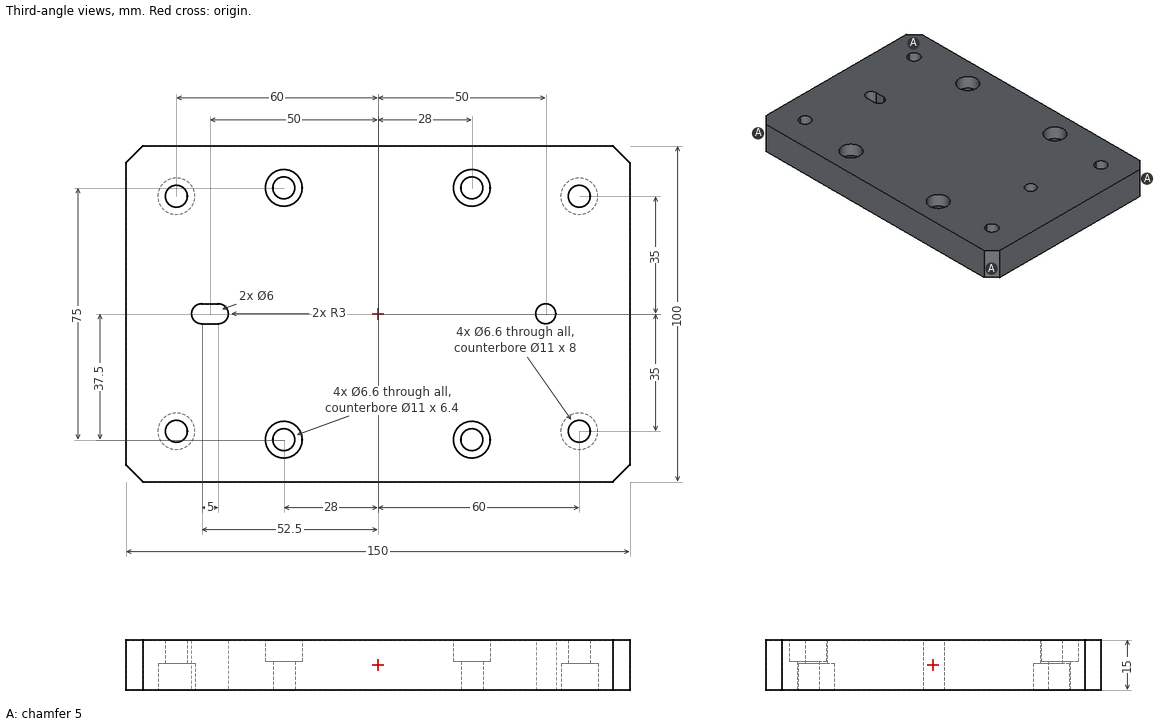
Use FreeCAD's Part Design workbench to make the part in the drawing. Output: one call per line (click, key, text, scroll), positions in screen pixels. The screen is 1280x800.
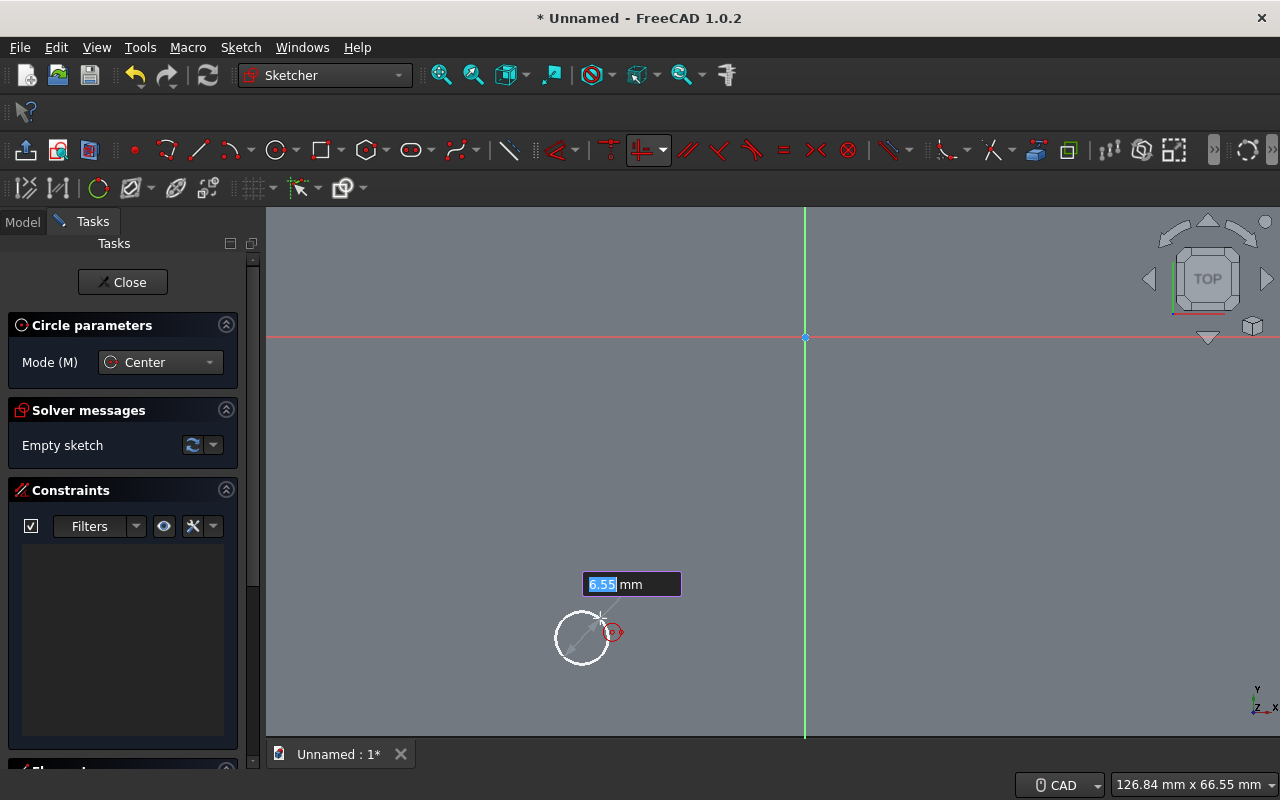
text(6.6)
key(Return)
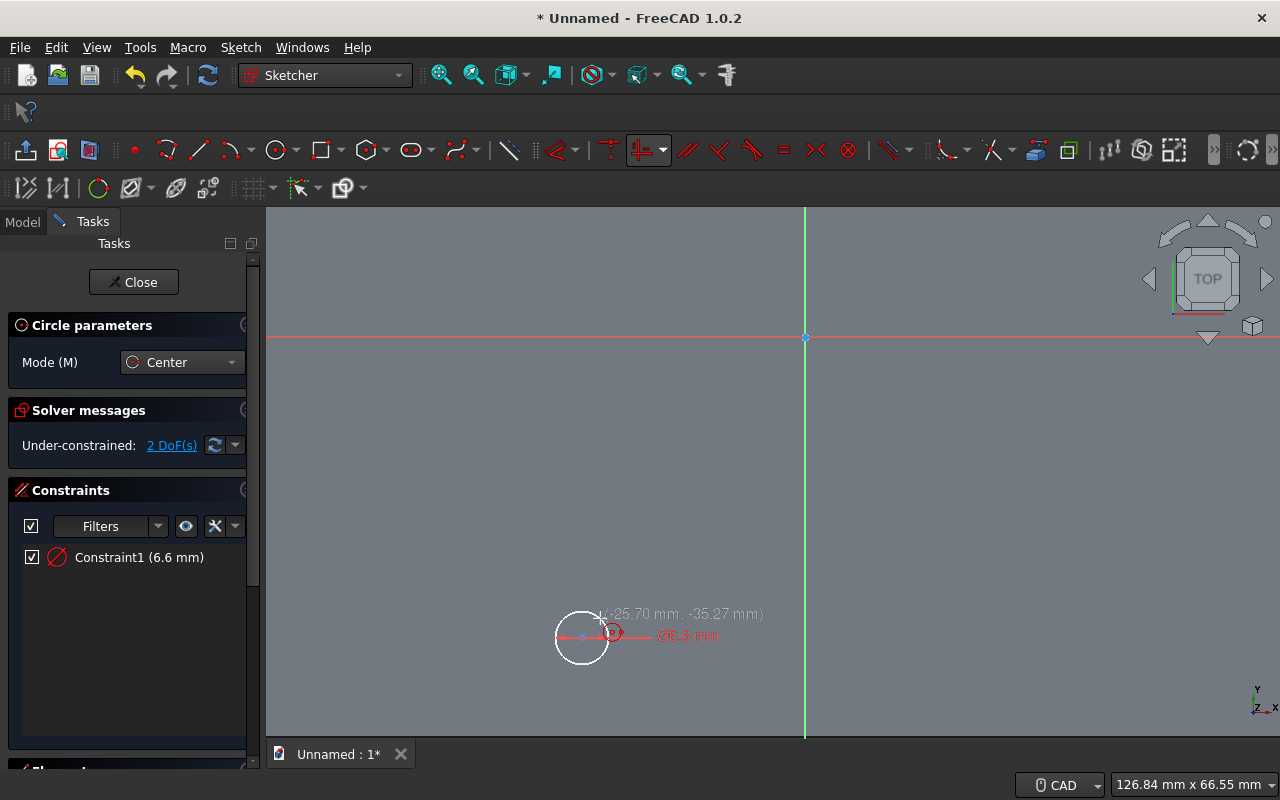
scroll(582, 638, down, 3)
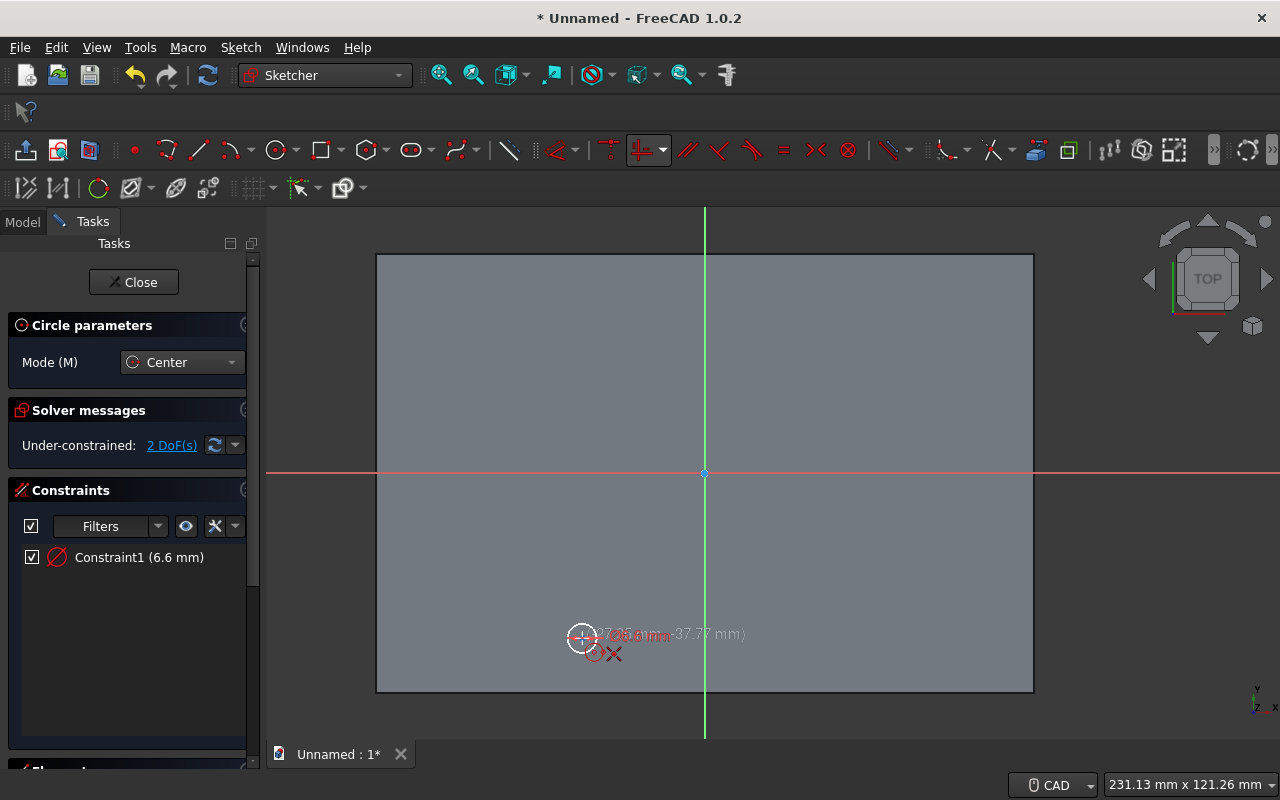
scroll(582, 309, up, 3)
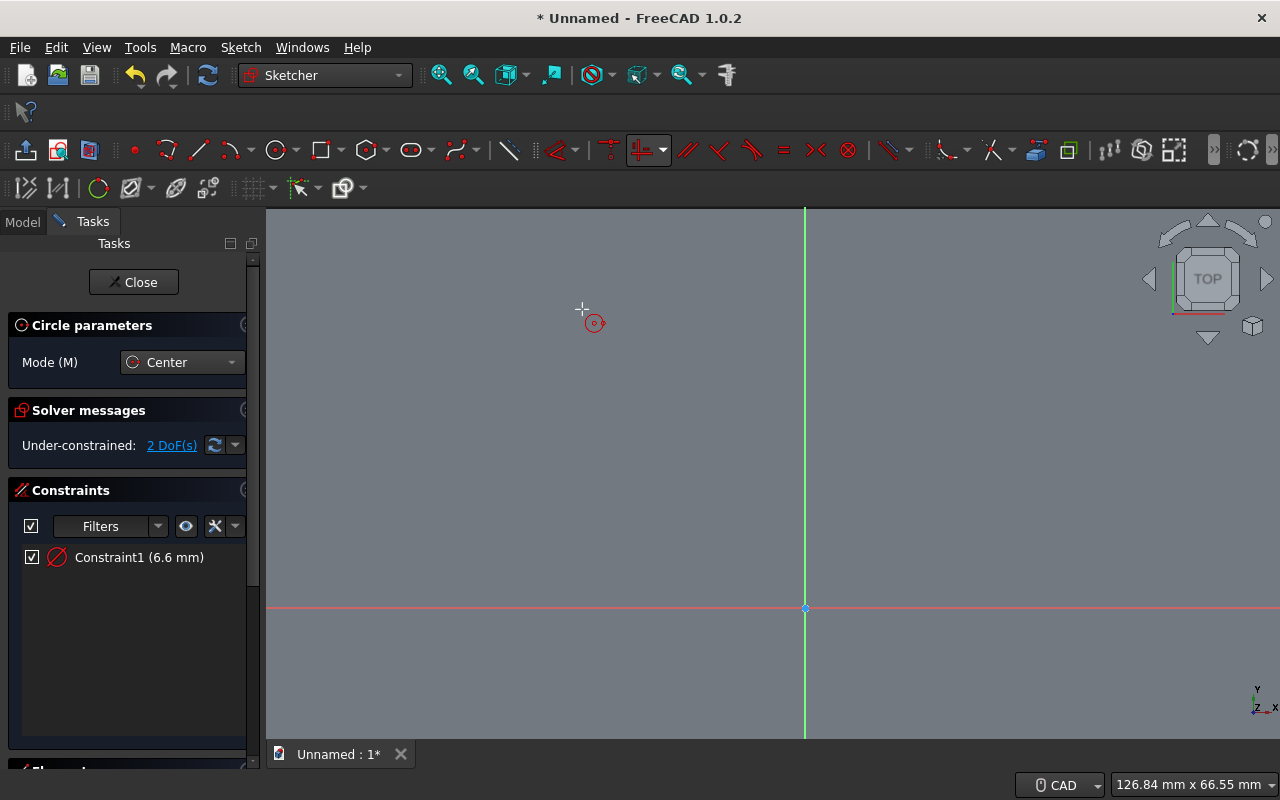
click(582, 308)
move(600, 290)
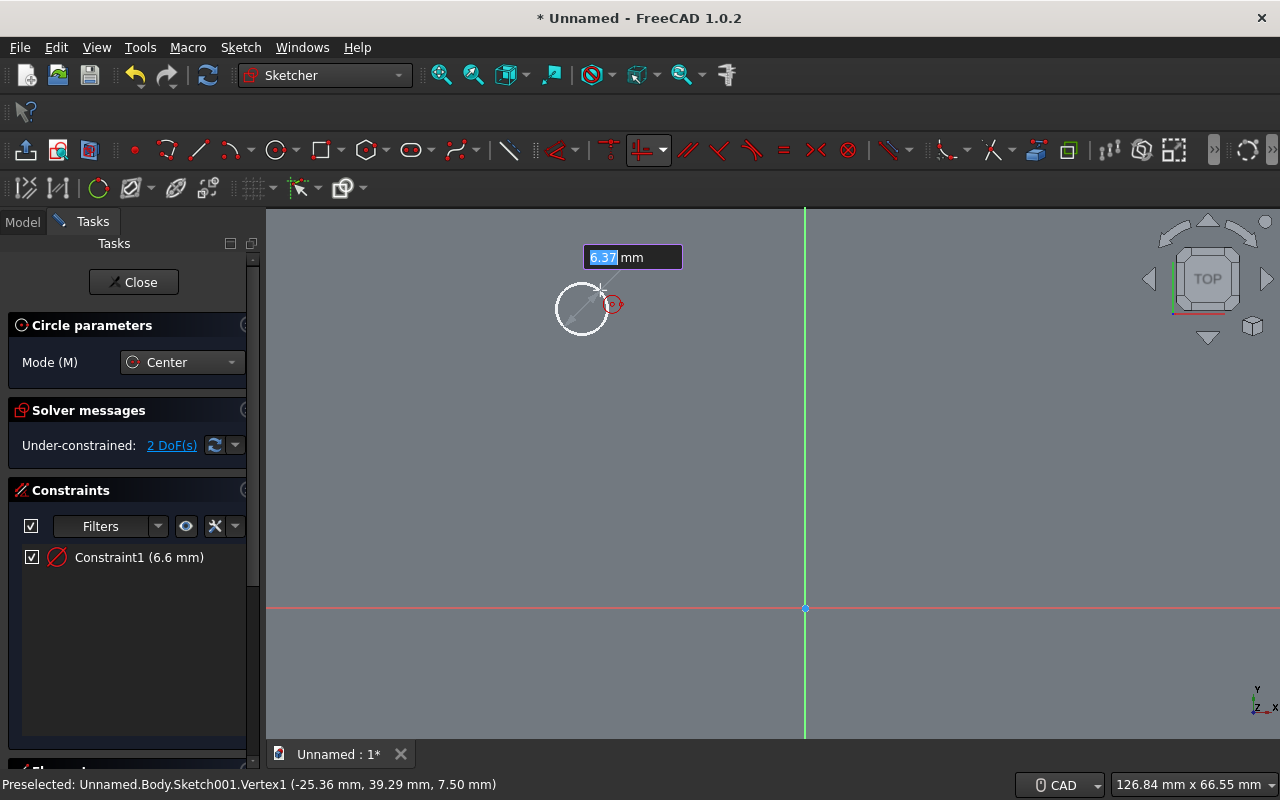
text(6.6)
key(Return)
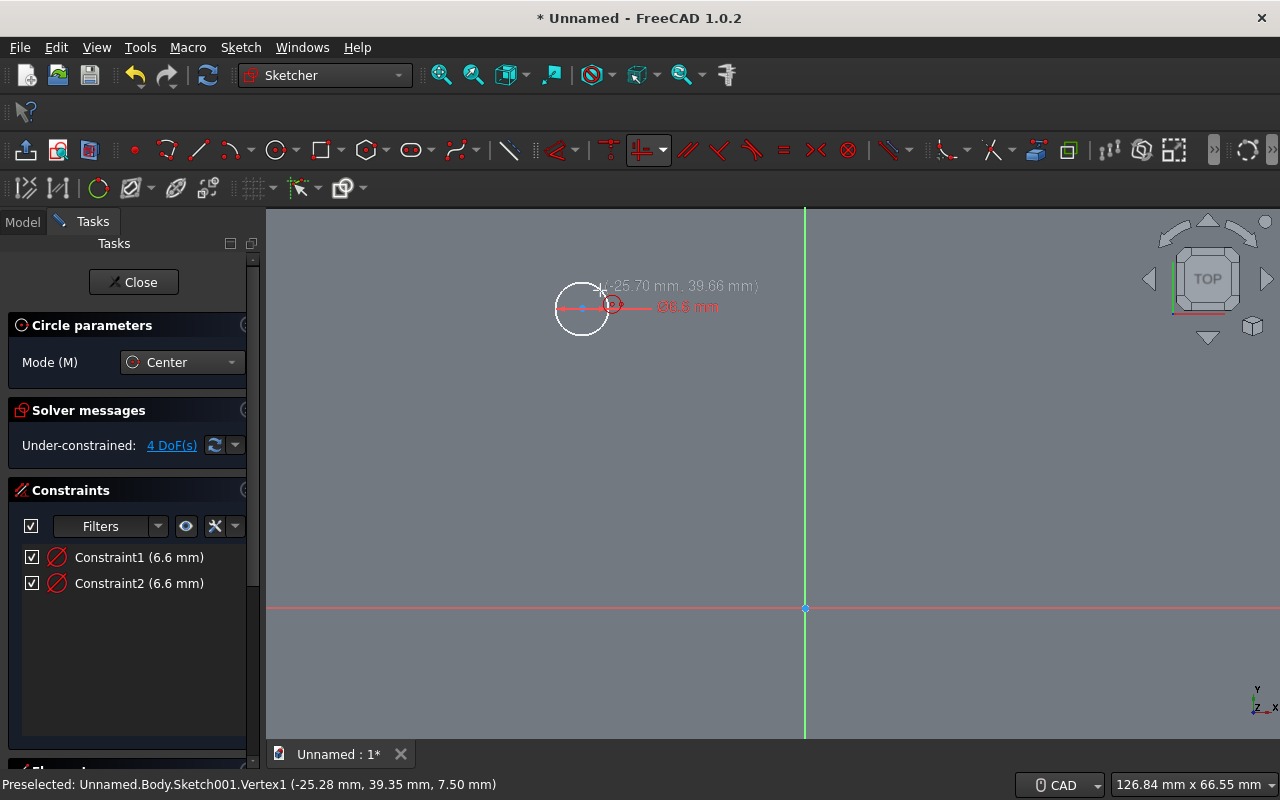
click(1029, 308)
move(1048, 290)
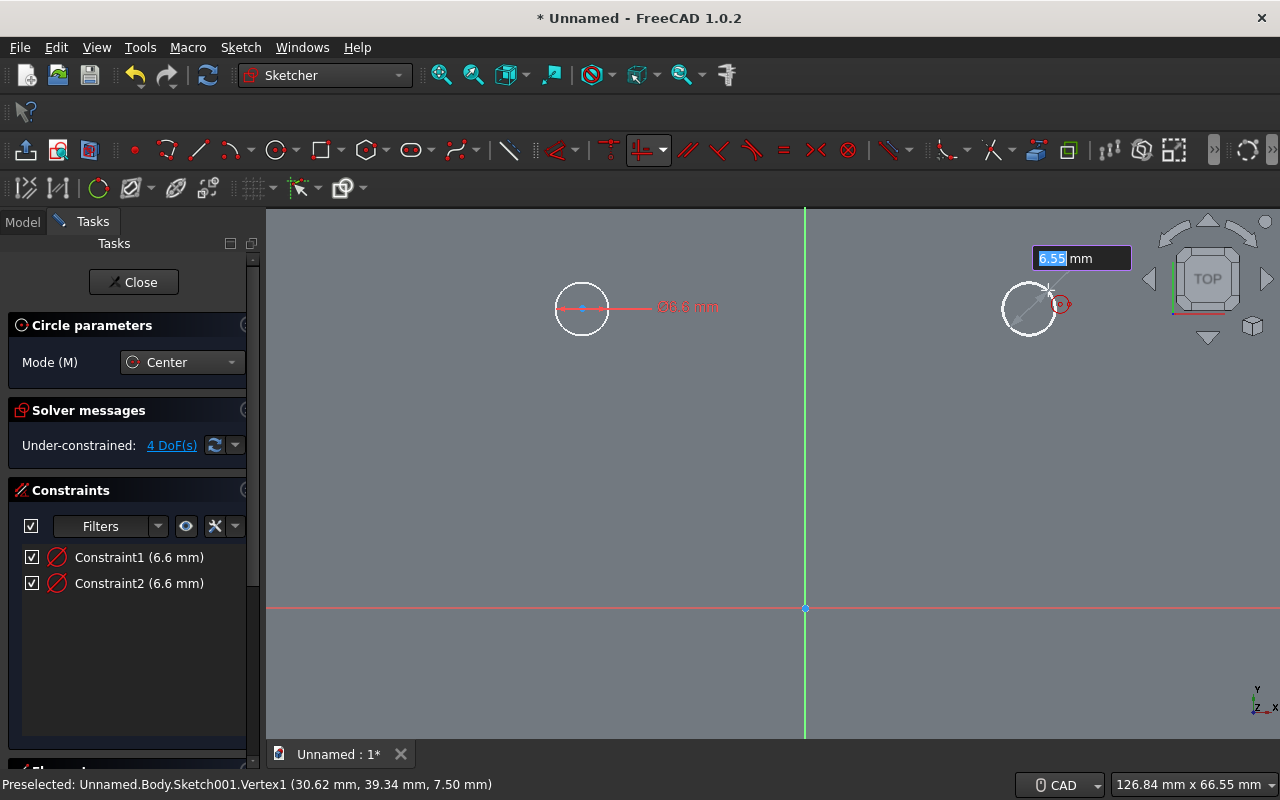
text(6.6)
key(Return)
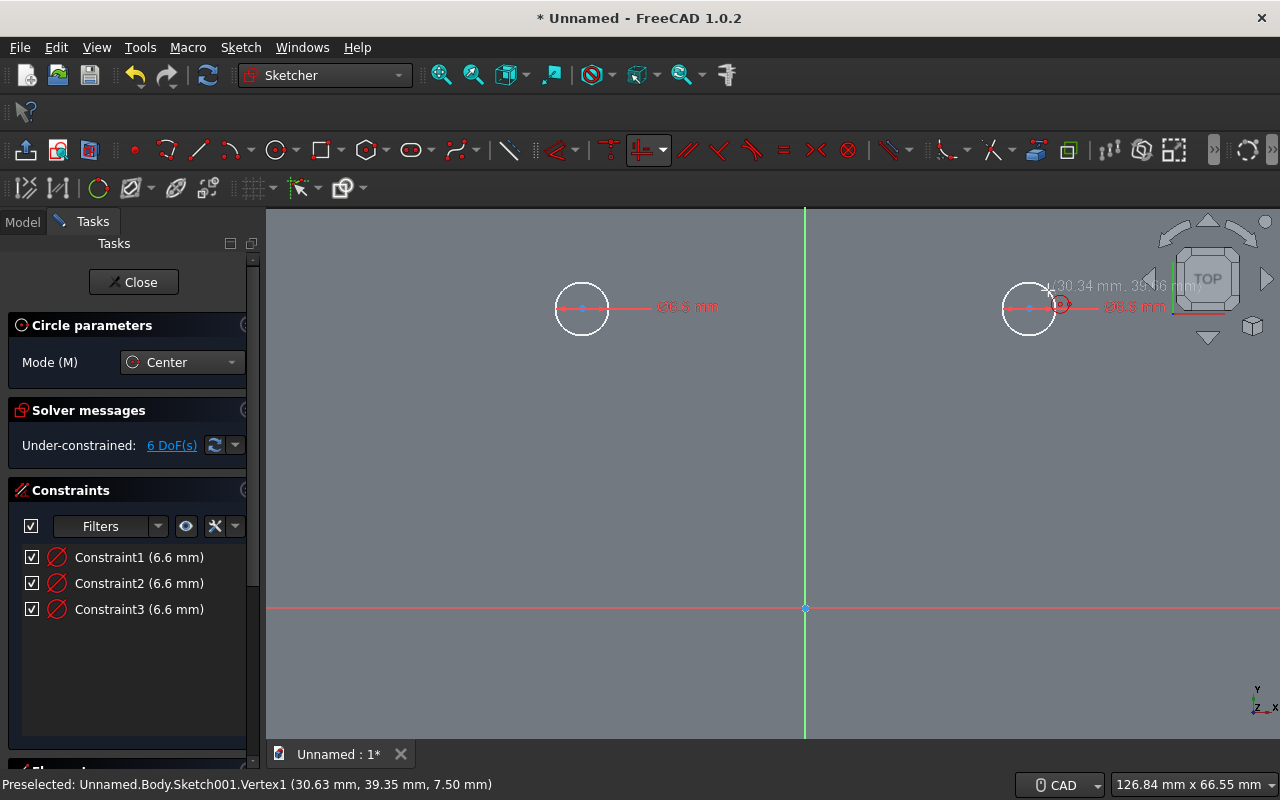
scroll(582, 309, down, 3)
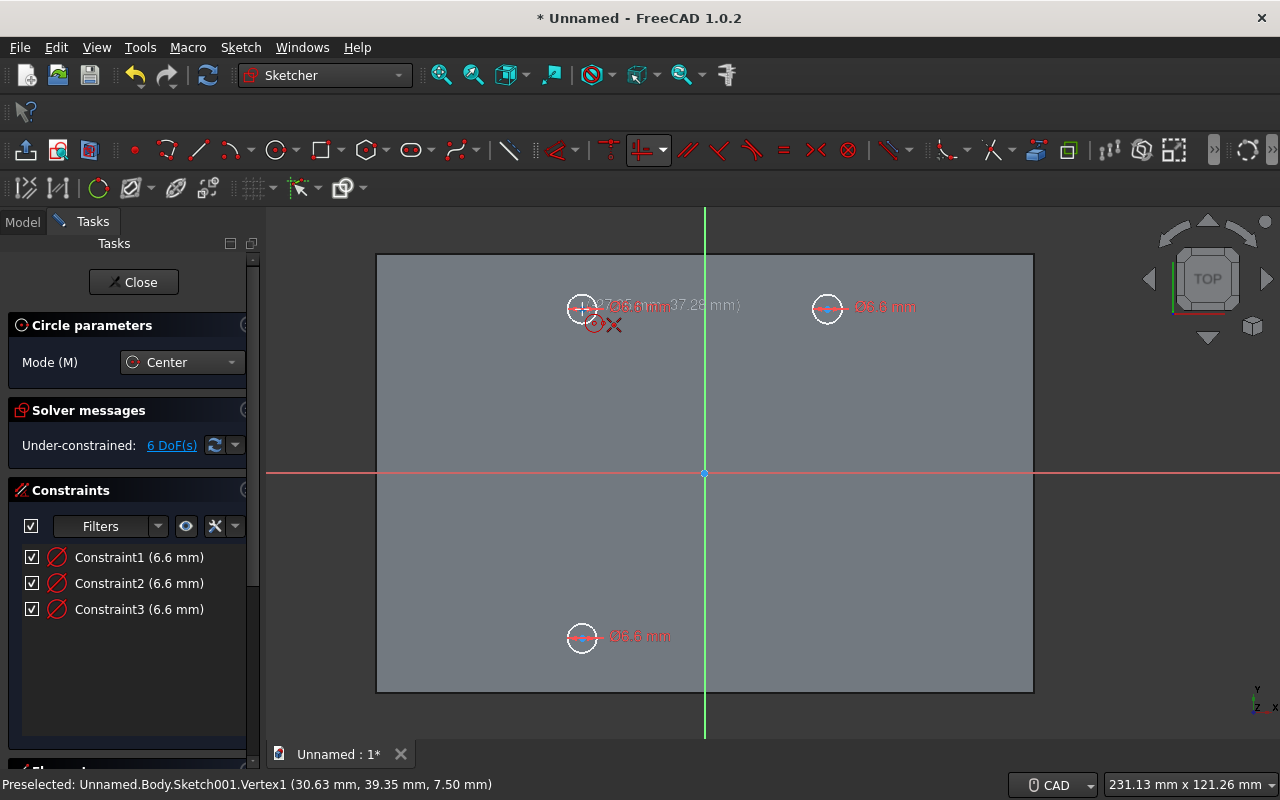
scroll(828, 638, up, 3)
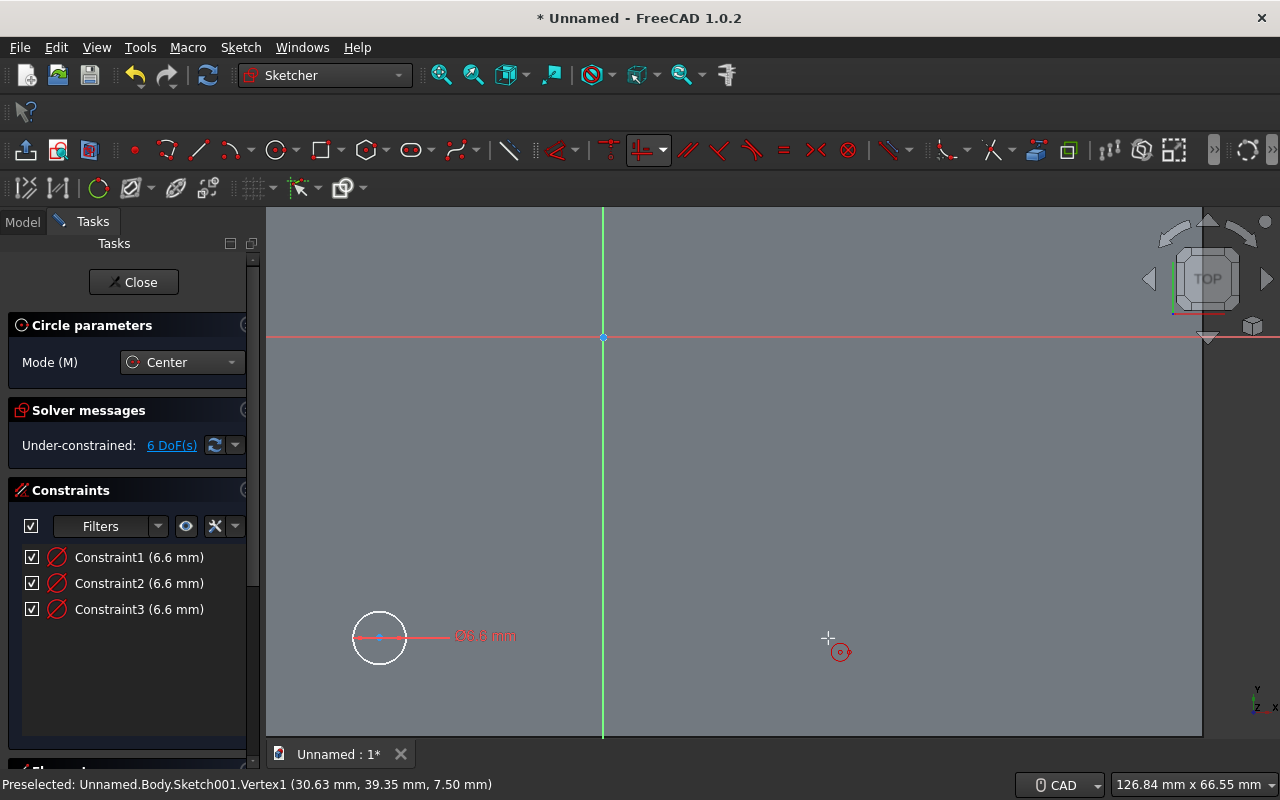
click(827, 637)
move(845, 618)